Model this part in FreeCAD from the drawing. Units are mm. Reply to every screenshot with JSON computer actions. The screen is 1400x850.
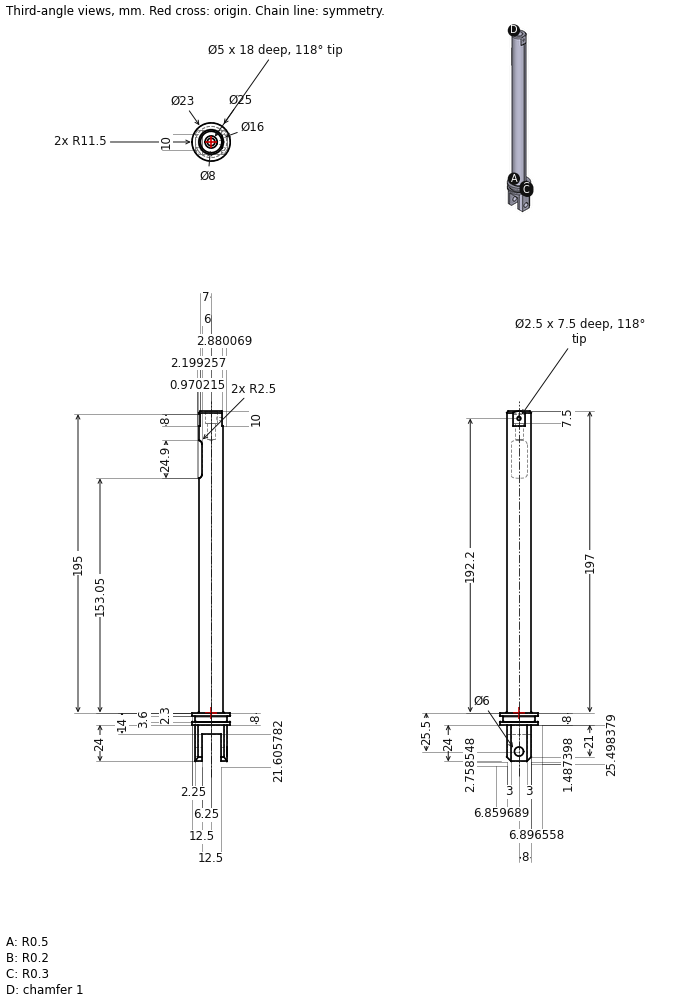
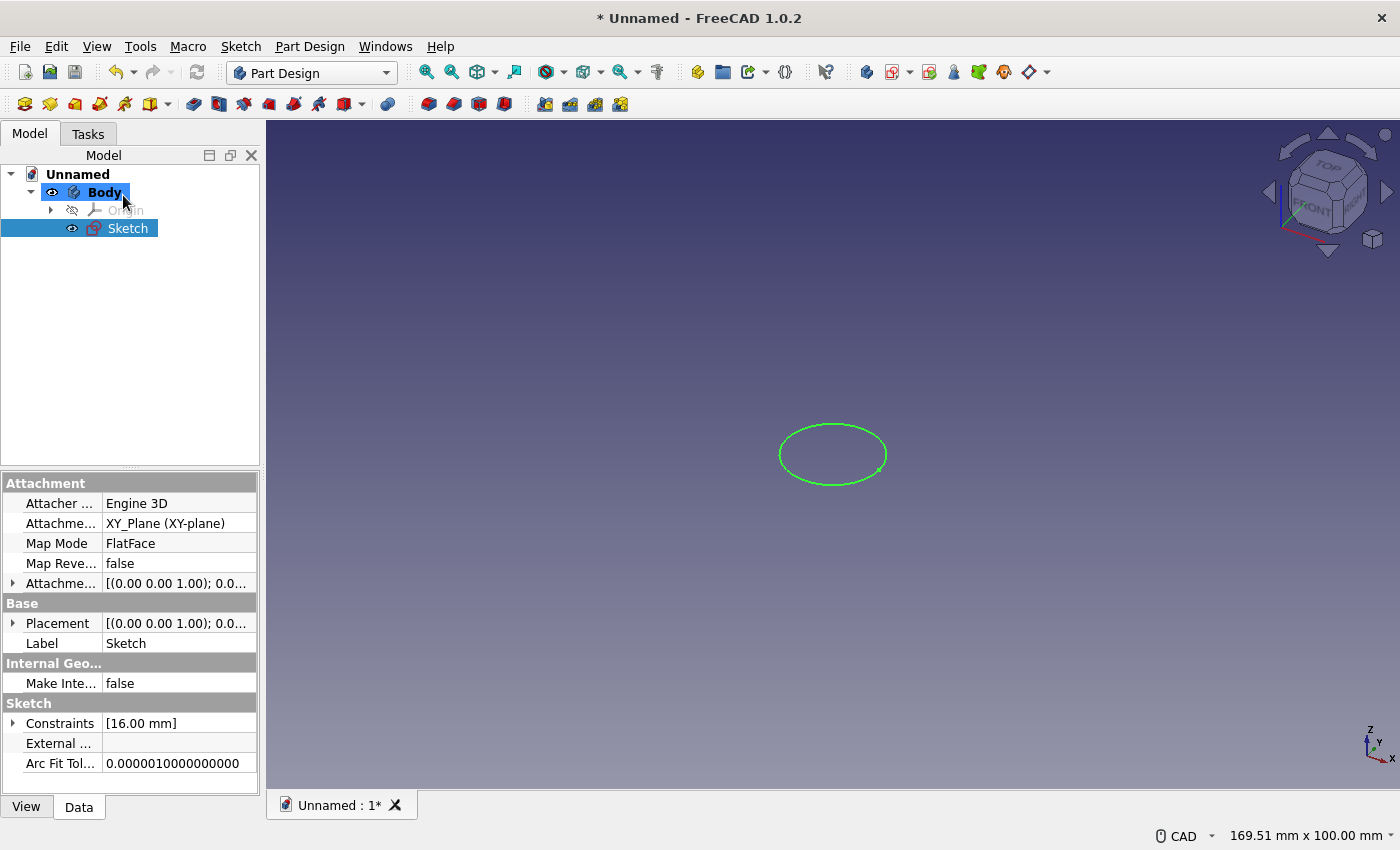
{"action": "left_click", "coordinate": [25, 104]}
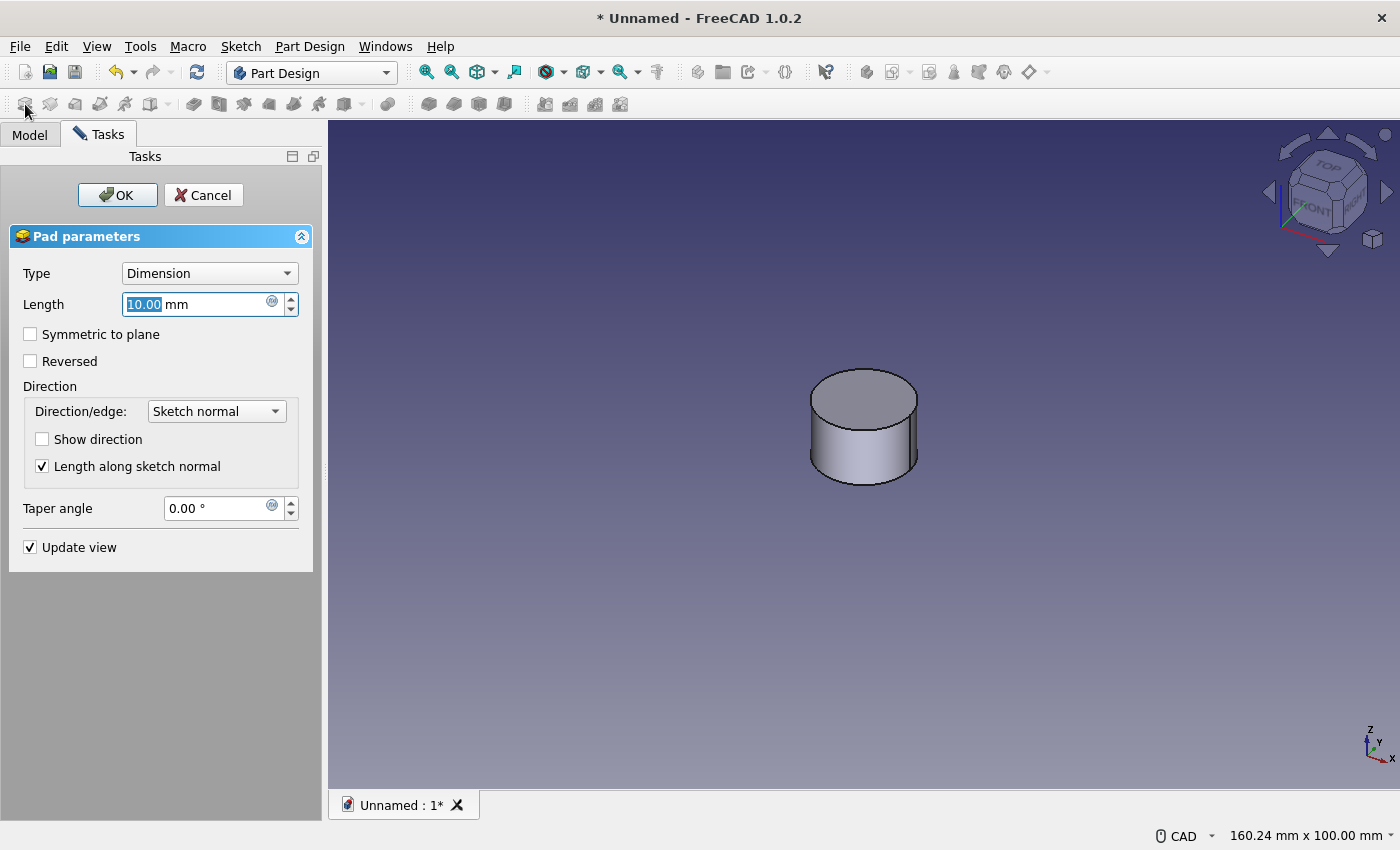
{"action": "type", "text": "197"}
{"action": "key", "text": "Tab"}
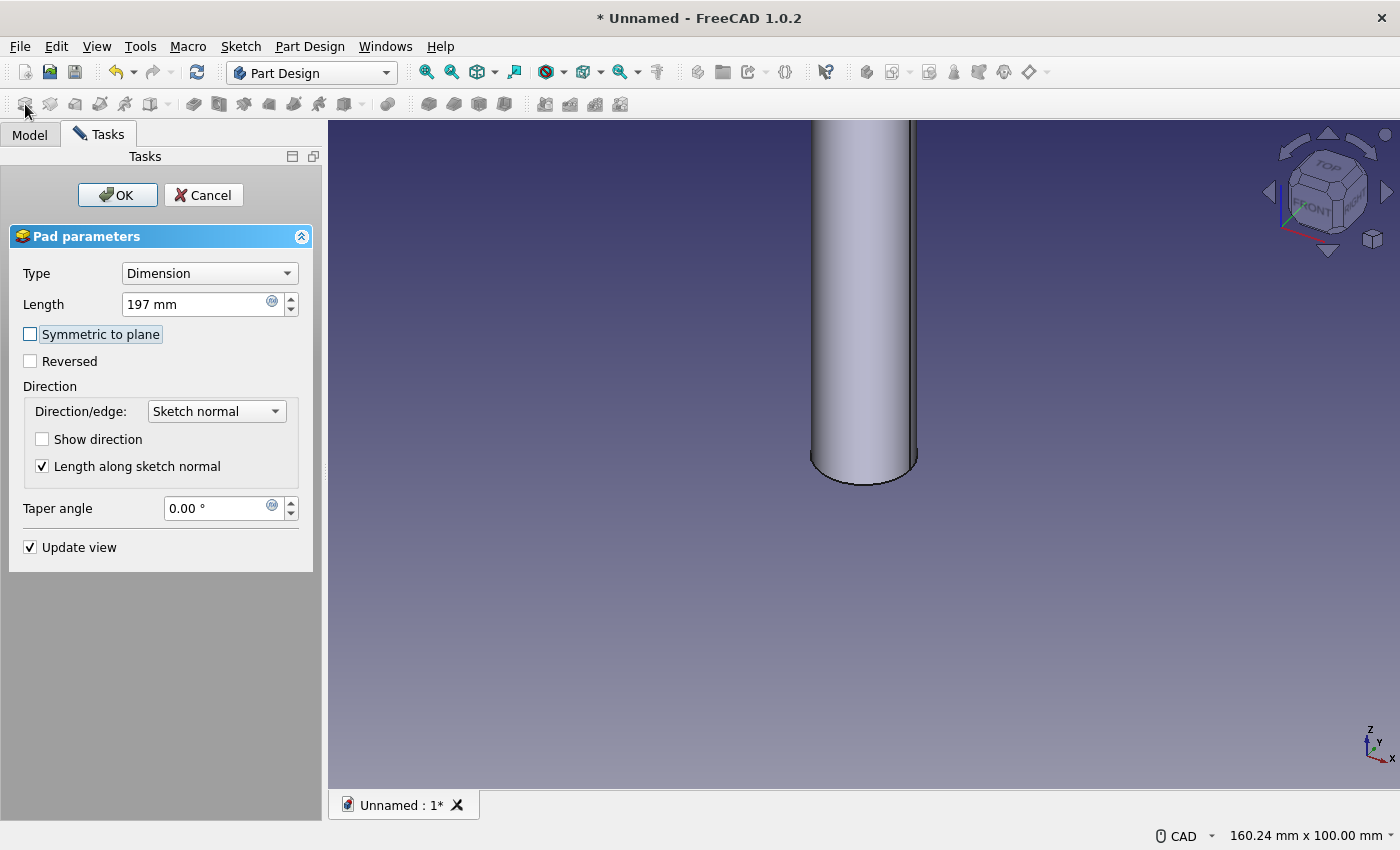
{"action": "left_click", "coordinate": [118, 195]}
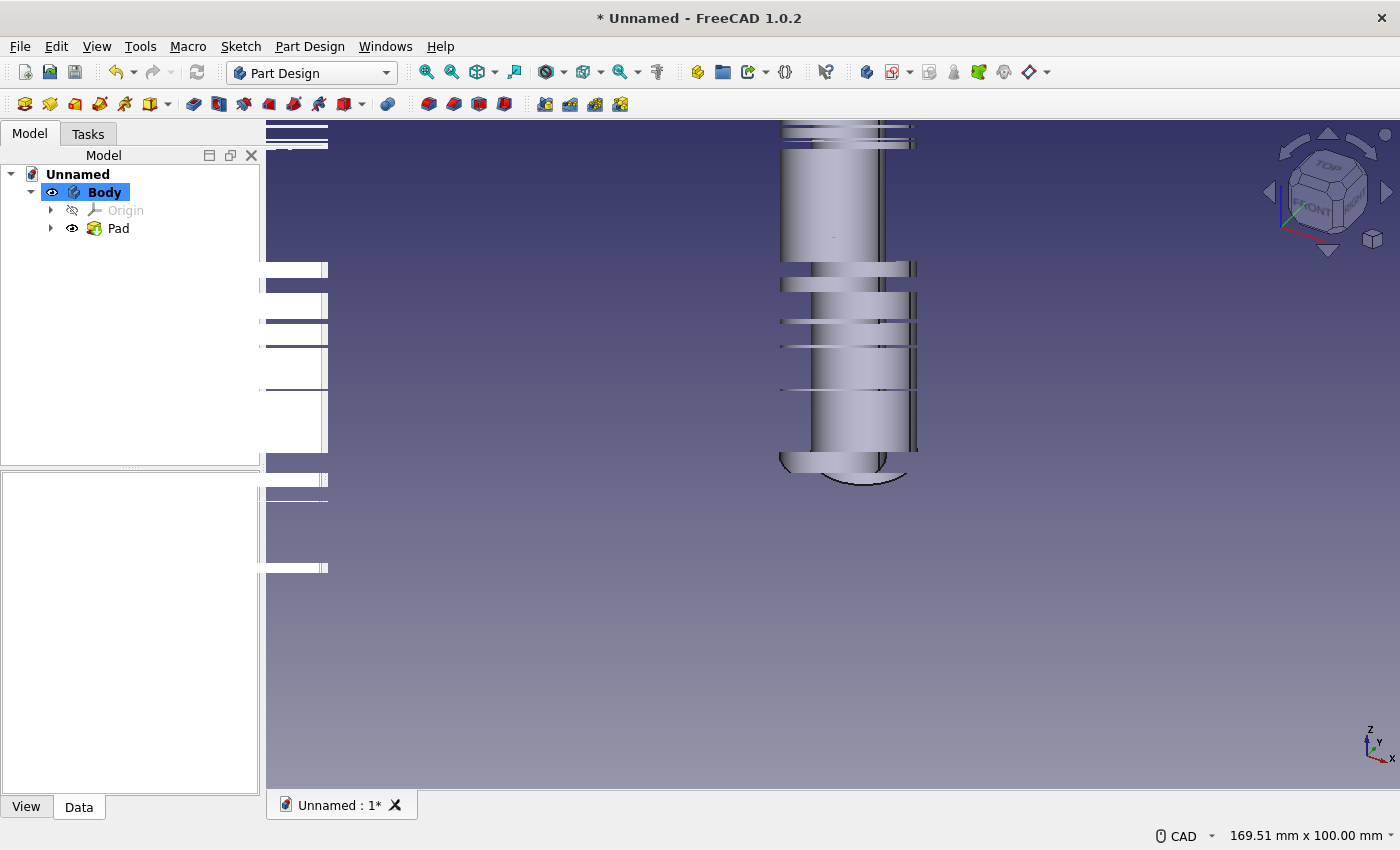
{"action": "left_click", "coordinate": [427, 72]}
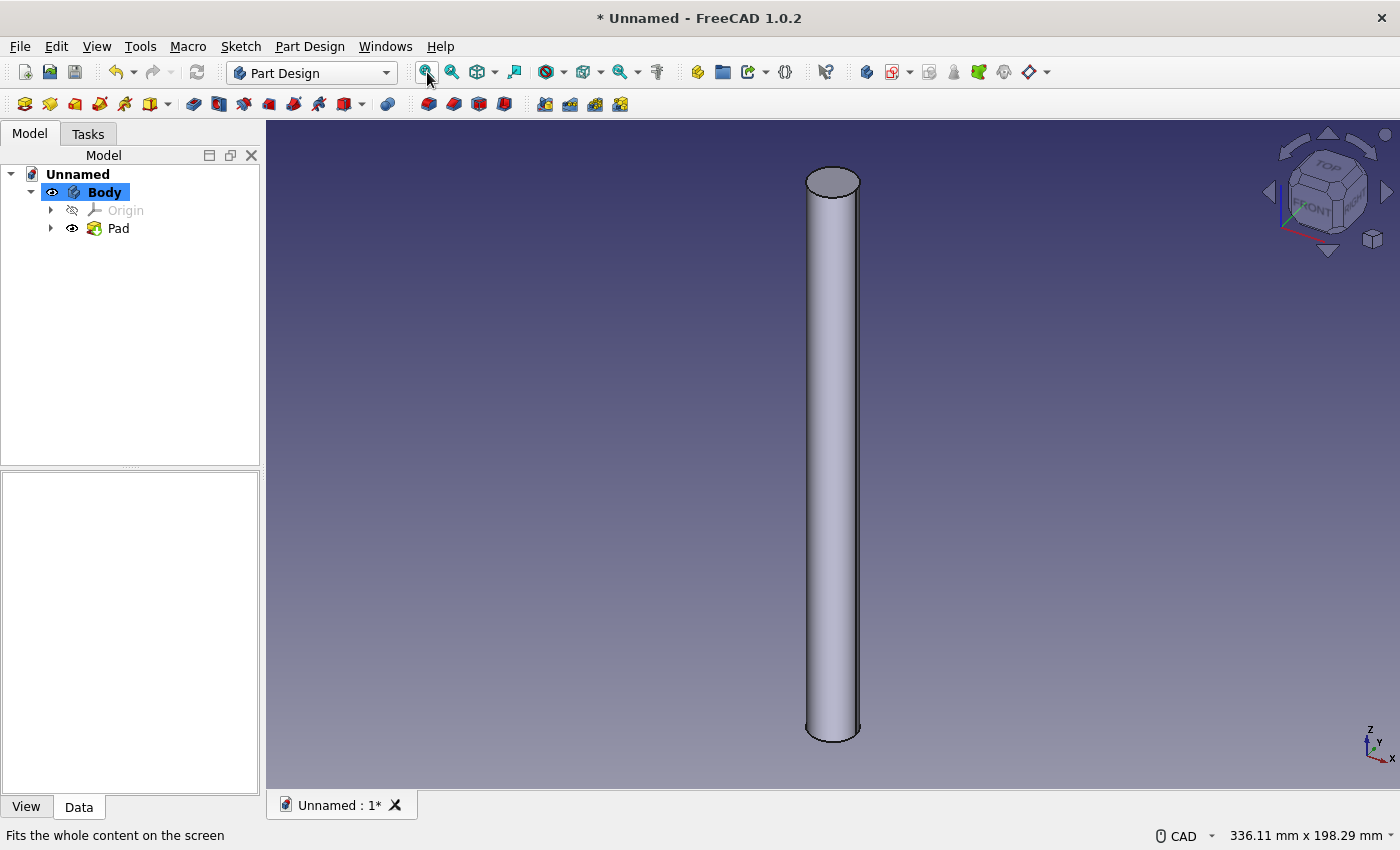
{"action": "key", "text": "5"}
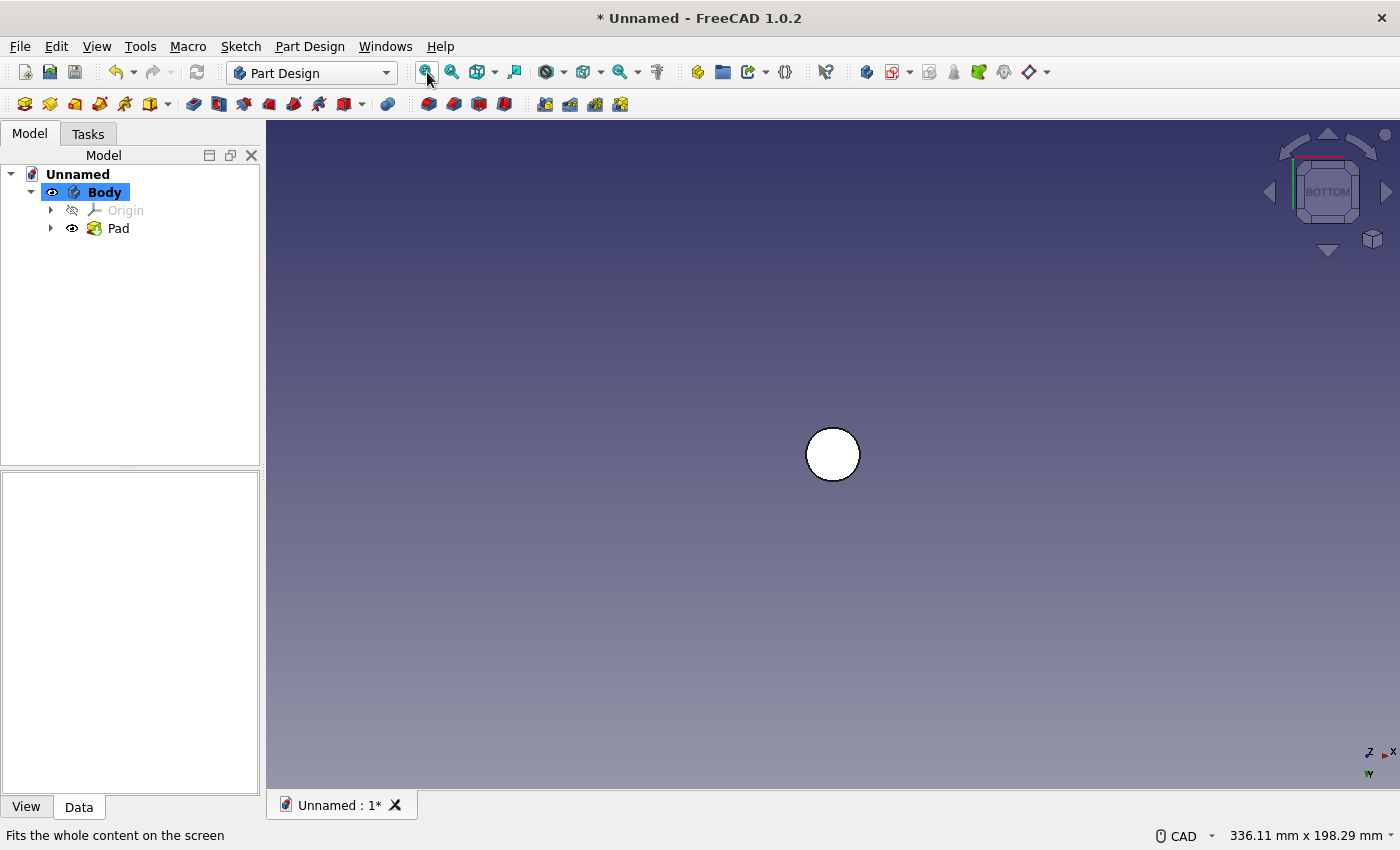
{"action": "left_click", "coordinate": [427, 72]}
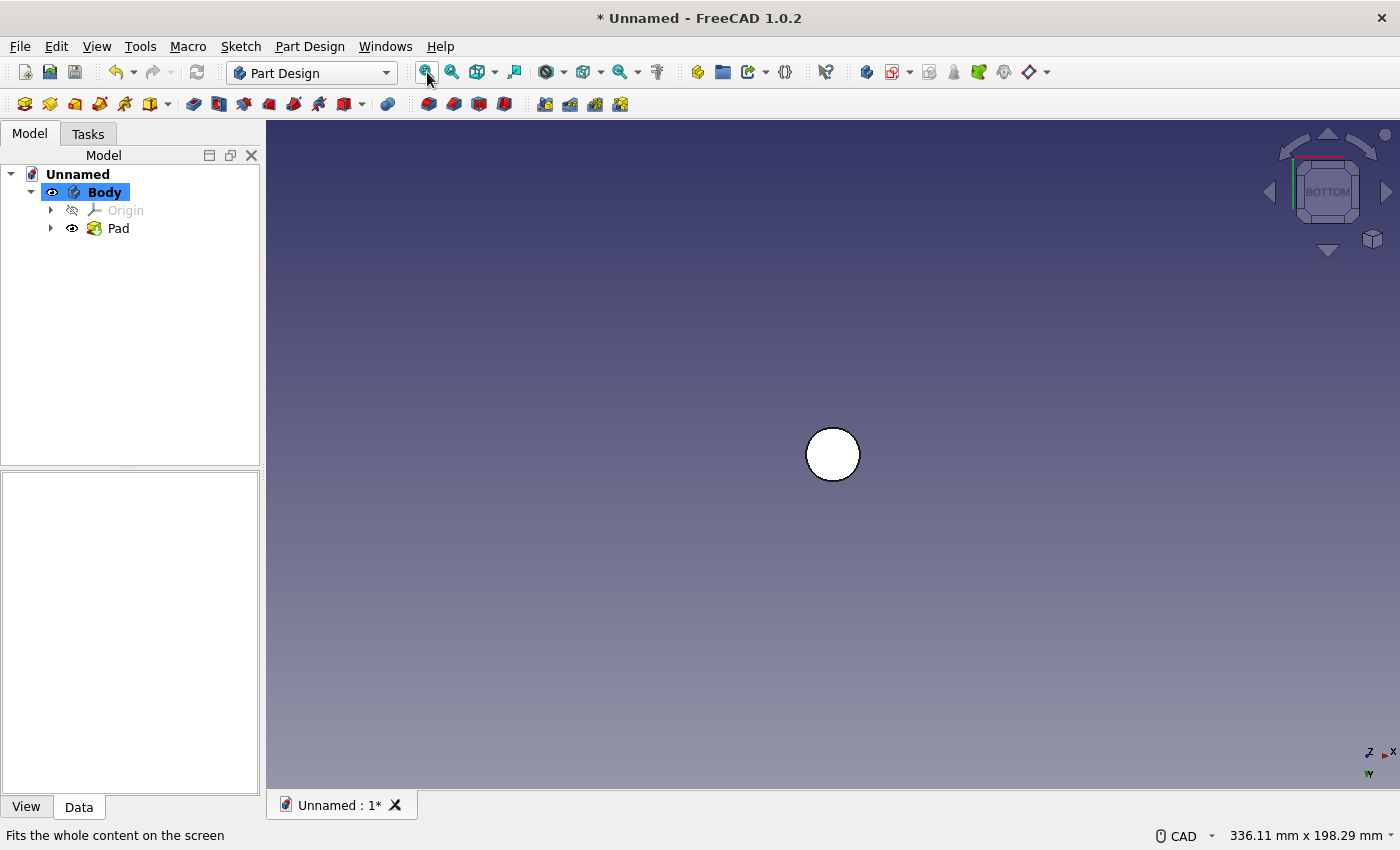
{"action": "left_click", "coordinate": [833, 453]}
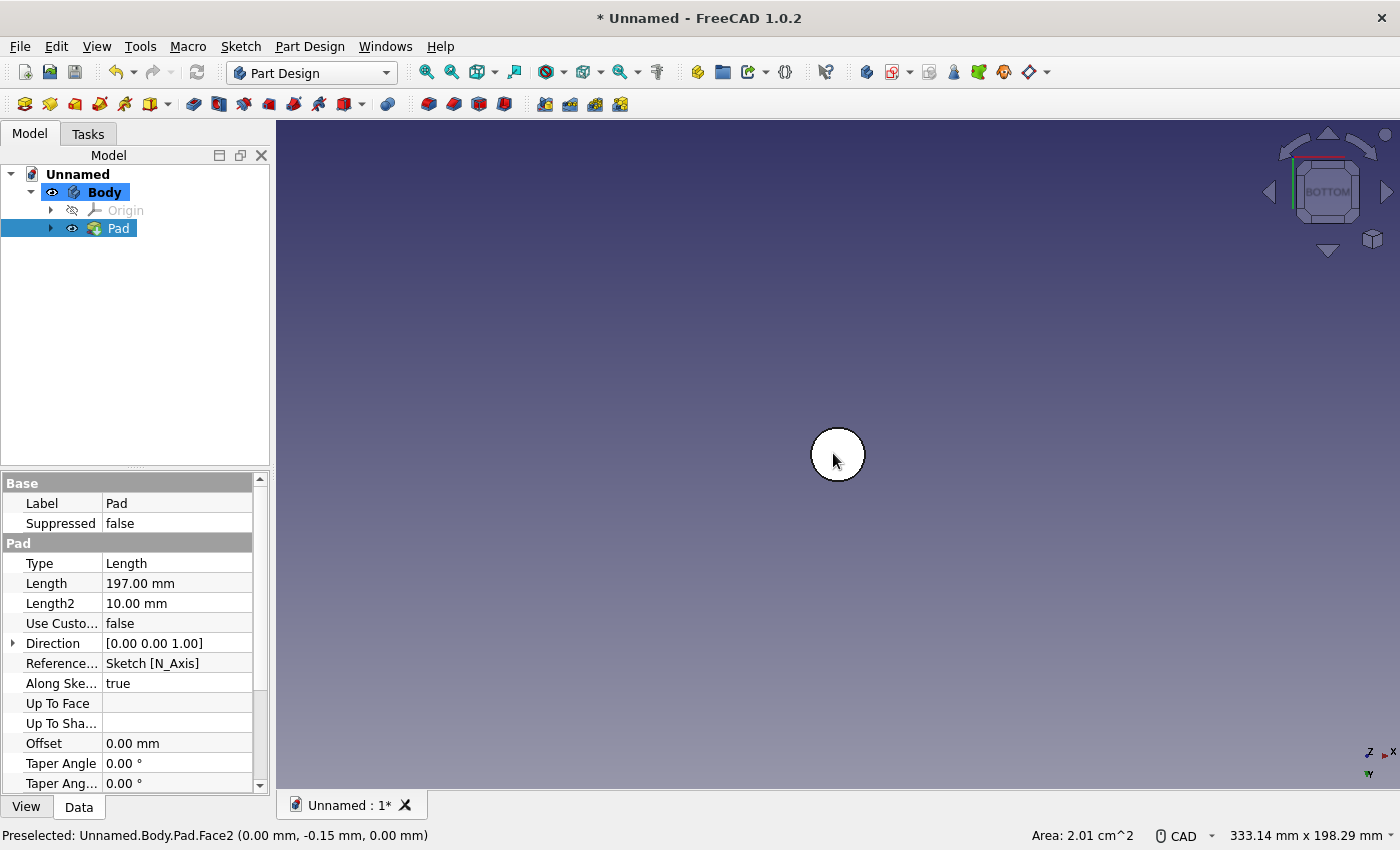
{"action": "left_click", "coordinate": [892, 72]}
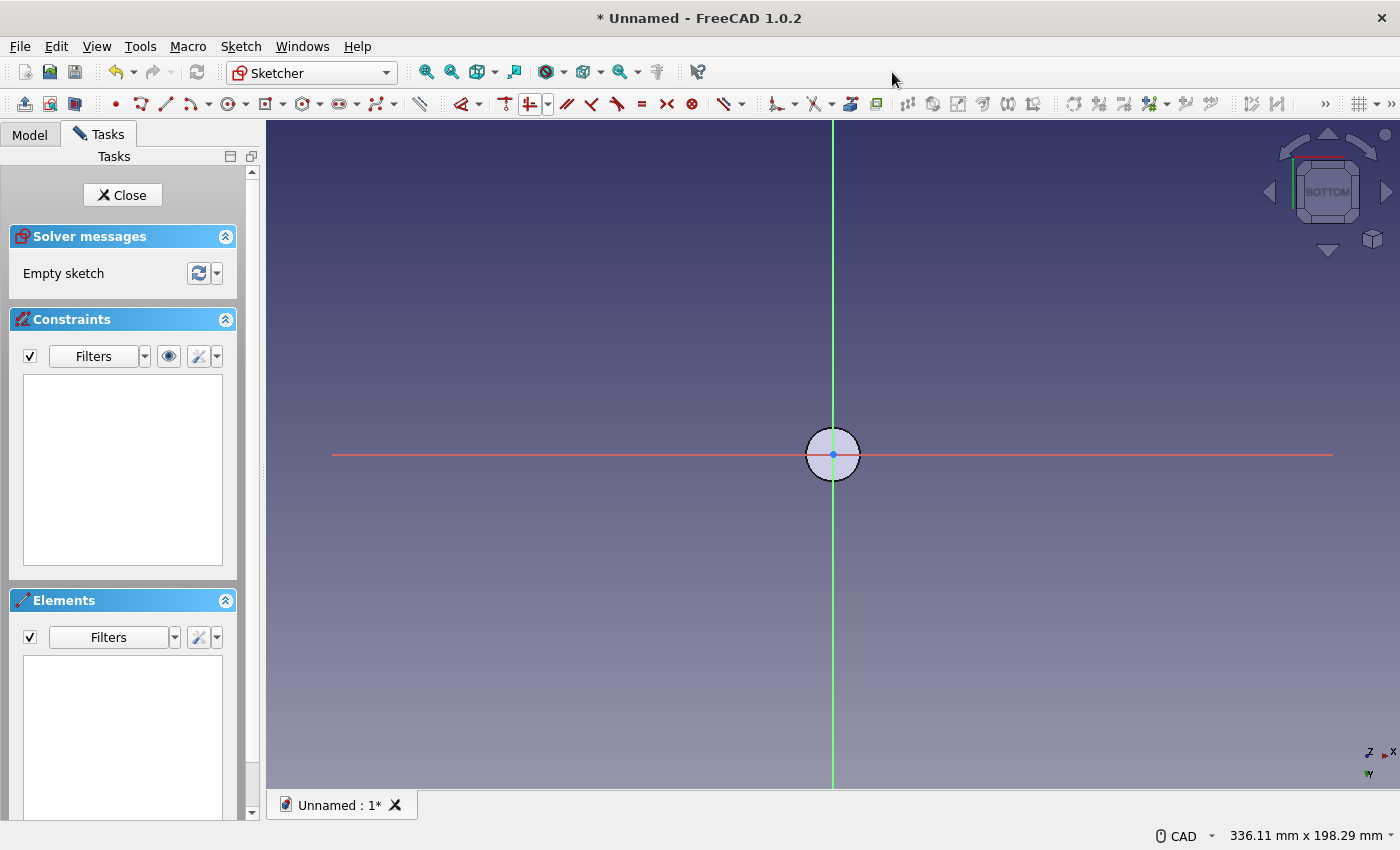
{"action": "scroll", "coordinate": [850, 454], "scroll_direction": "up", "scroll_amount": 8}